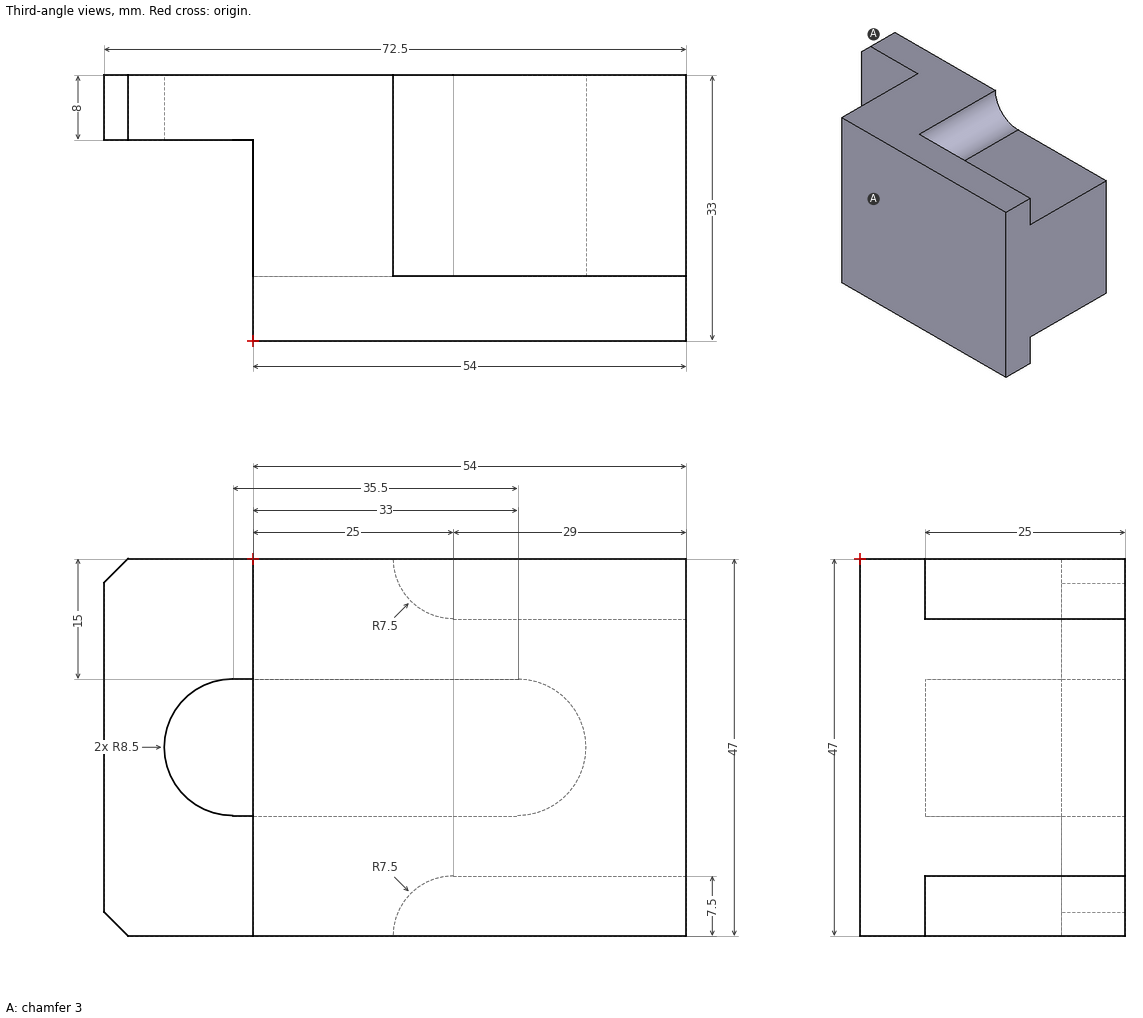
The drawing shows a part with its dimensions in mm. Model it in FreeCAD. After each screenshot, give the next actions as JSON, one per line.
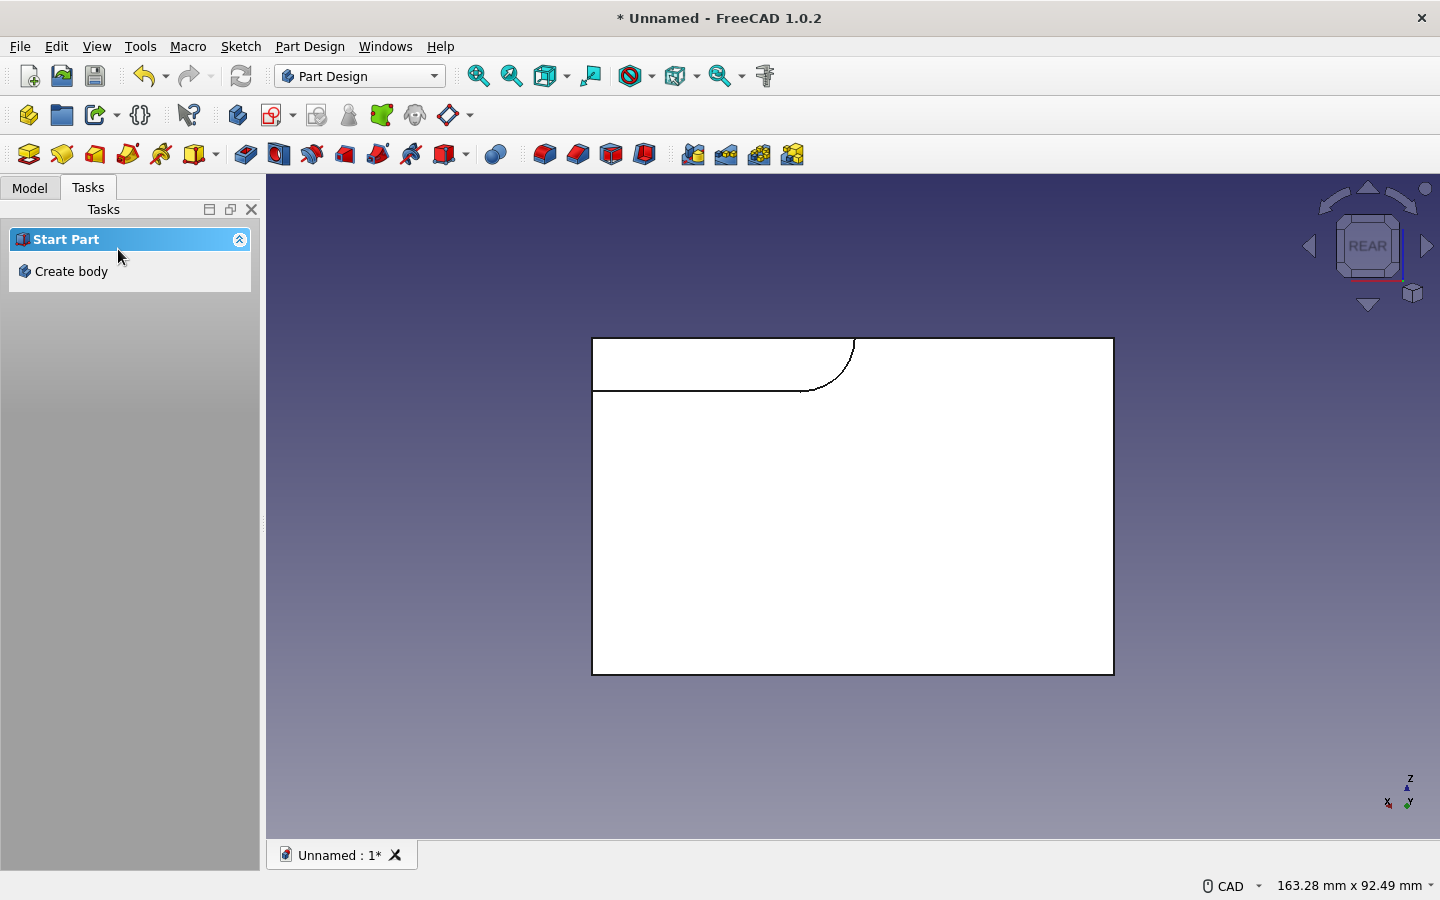
{"action": "left_click", "coordinate": [927, 505]}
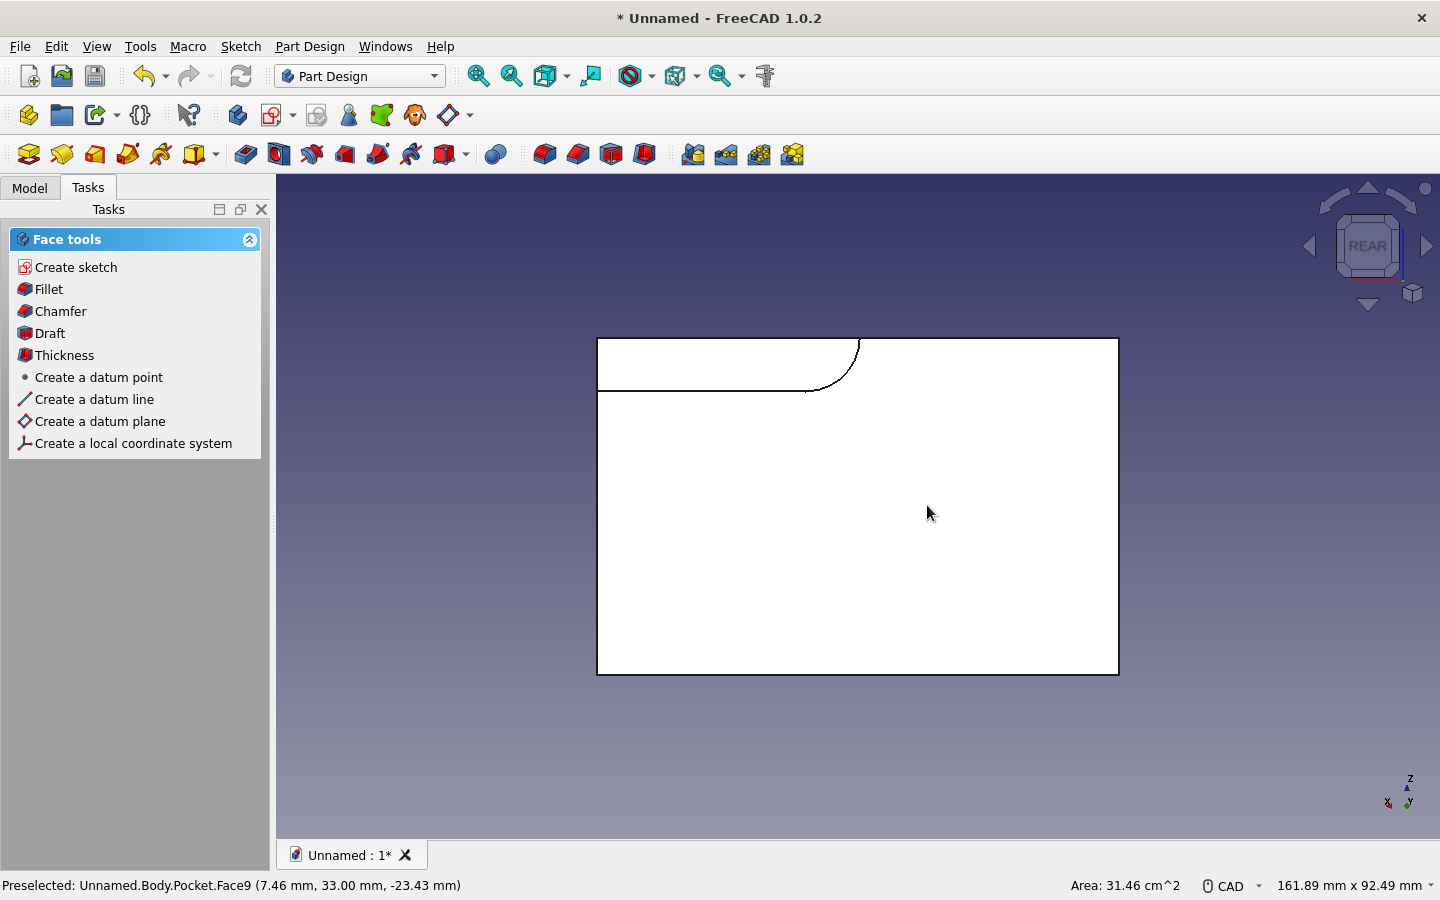
{"action": "left_click", "coordinate": [270, 116]}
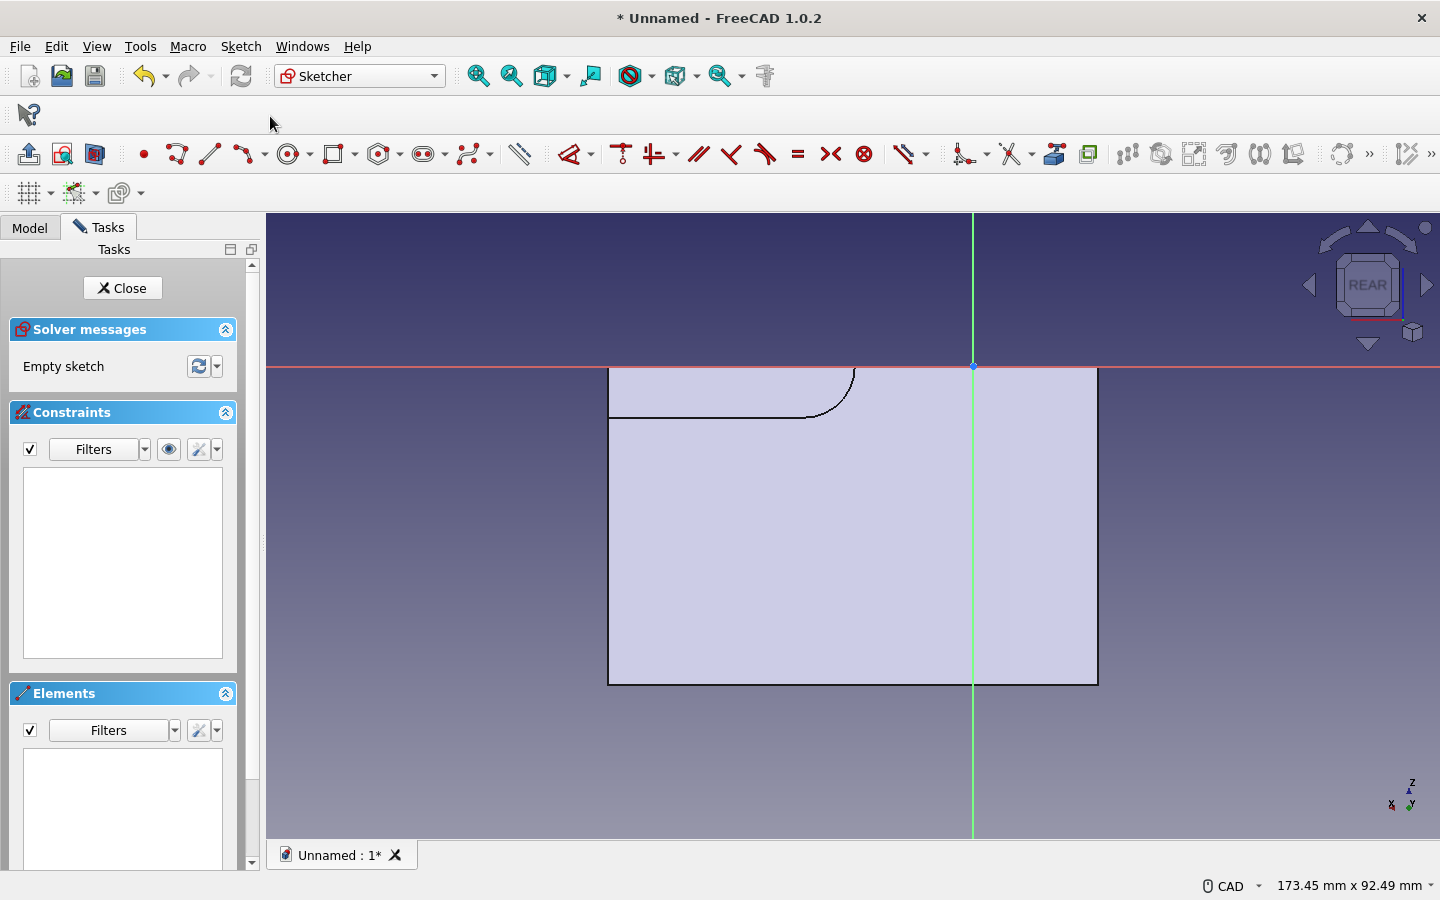
{"action": "key", "text": "g m"}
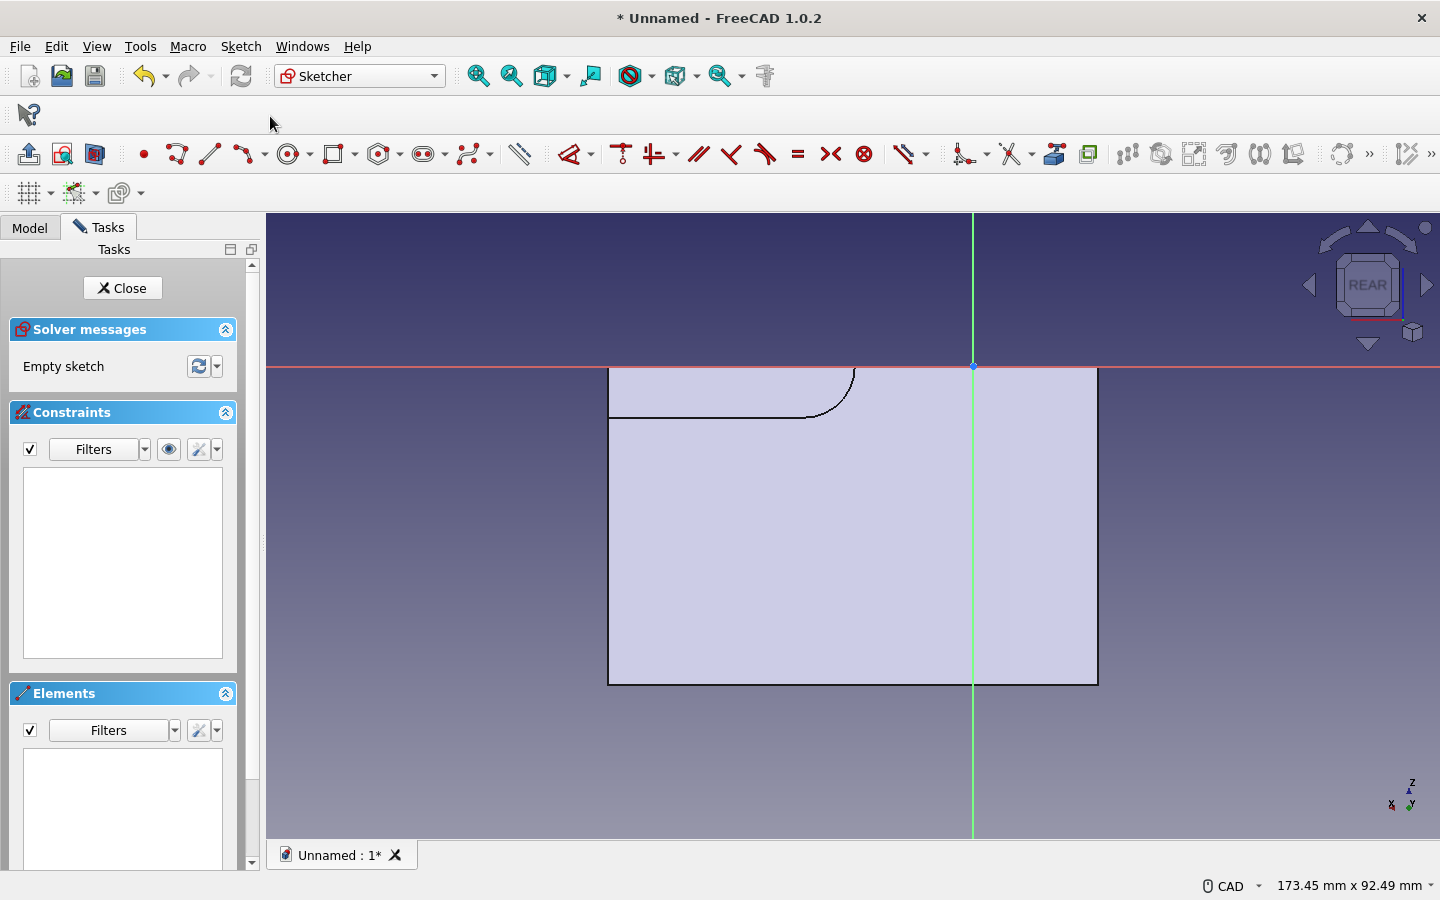
{"action": "left_click", "coordinate": [804, 634]}
{"action": "left_click", "coordinate": [608, 634]}
{"action": "left_click", "coordinate": [608, 685]}
{"action": "left_click", "coordinate": [855, 685]}
{"action": "right_click", "coordinate": [855, 685]}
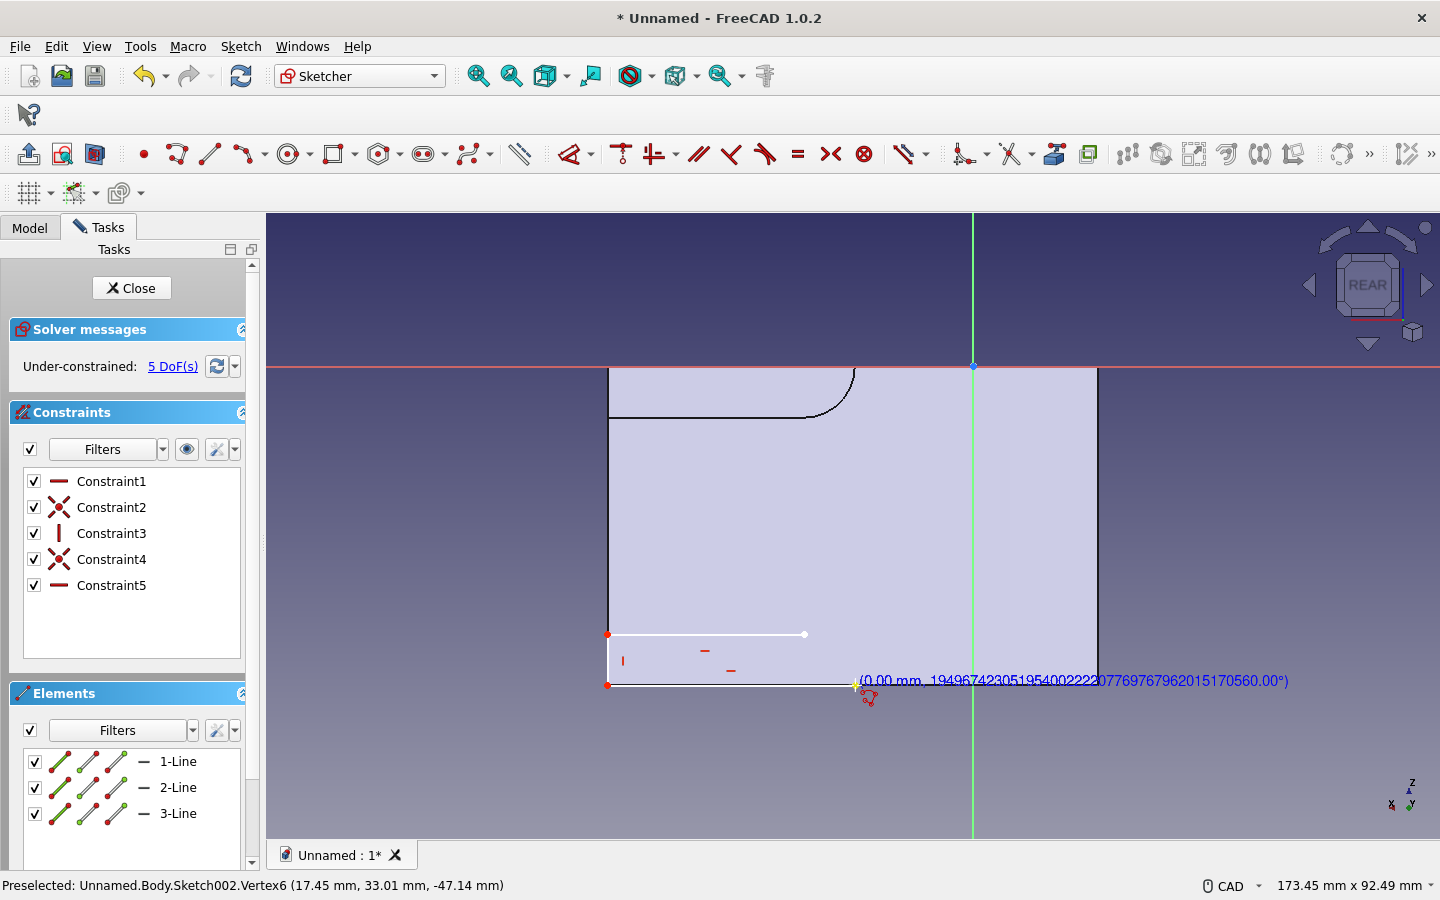
{"action": "key", "text": "g 3 a"}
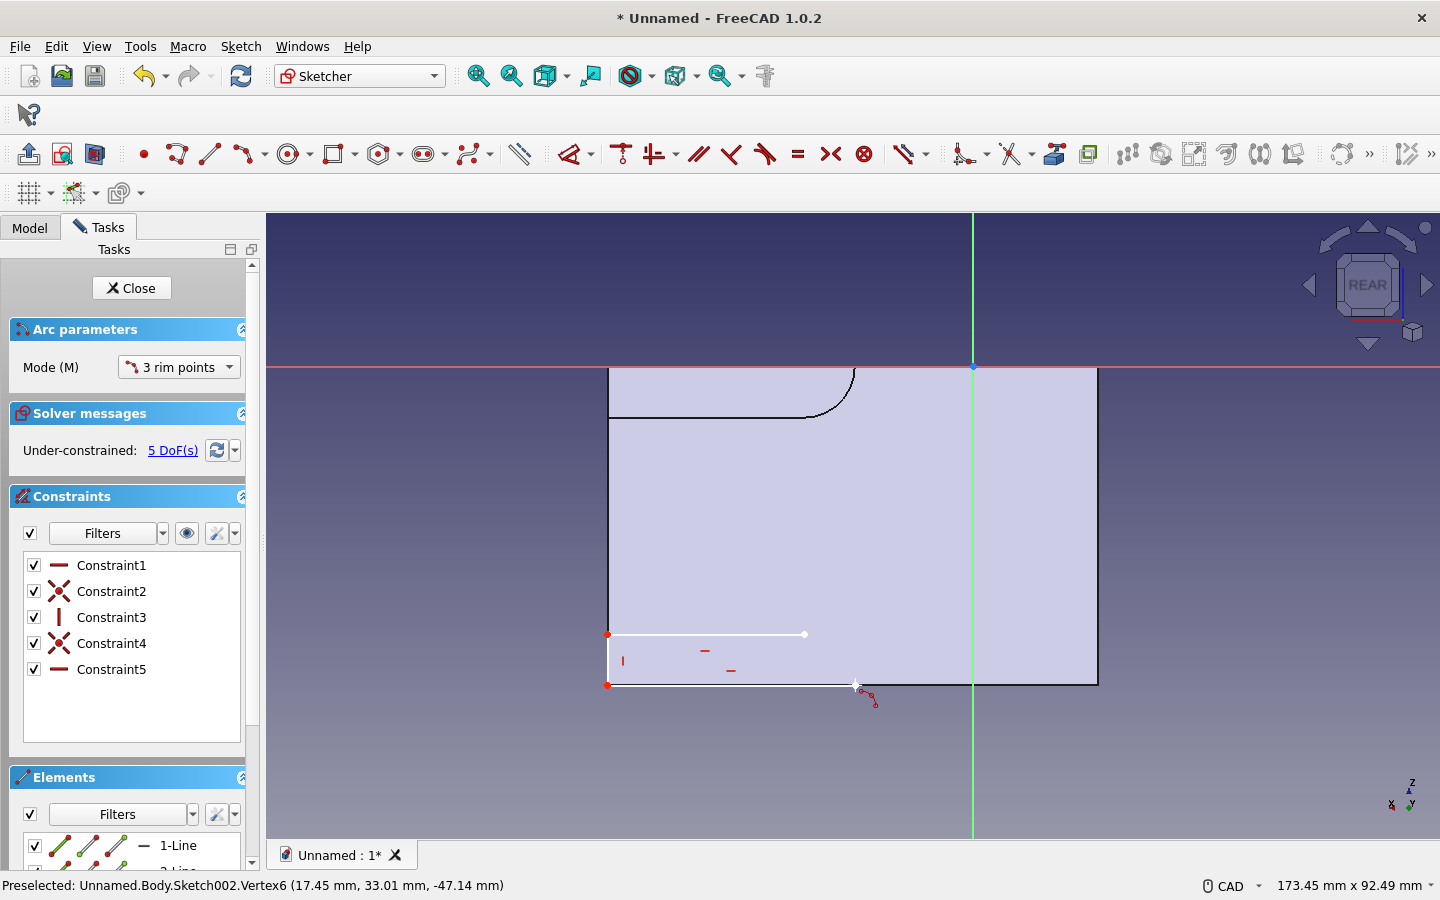
{"action": "left_click", "coordinate": [855, 686]}
{"action": "left_click", "coordinate": [804, 635]}
{"action": "left_click", "coordinate": [840, 649]}
{"action": "key", "text": "Escape"}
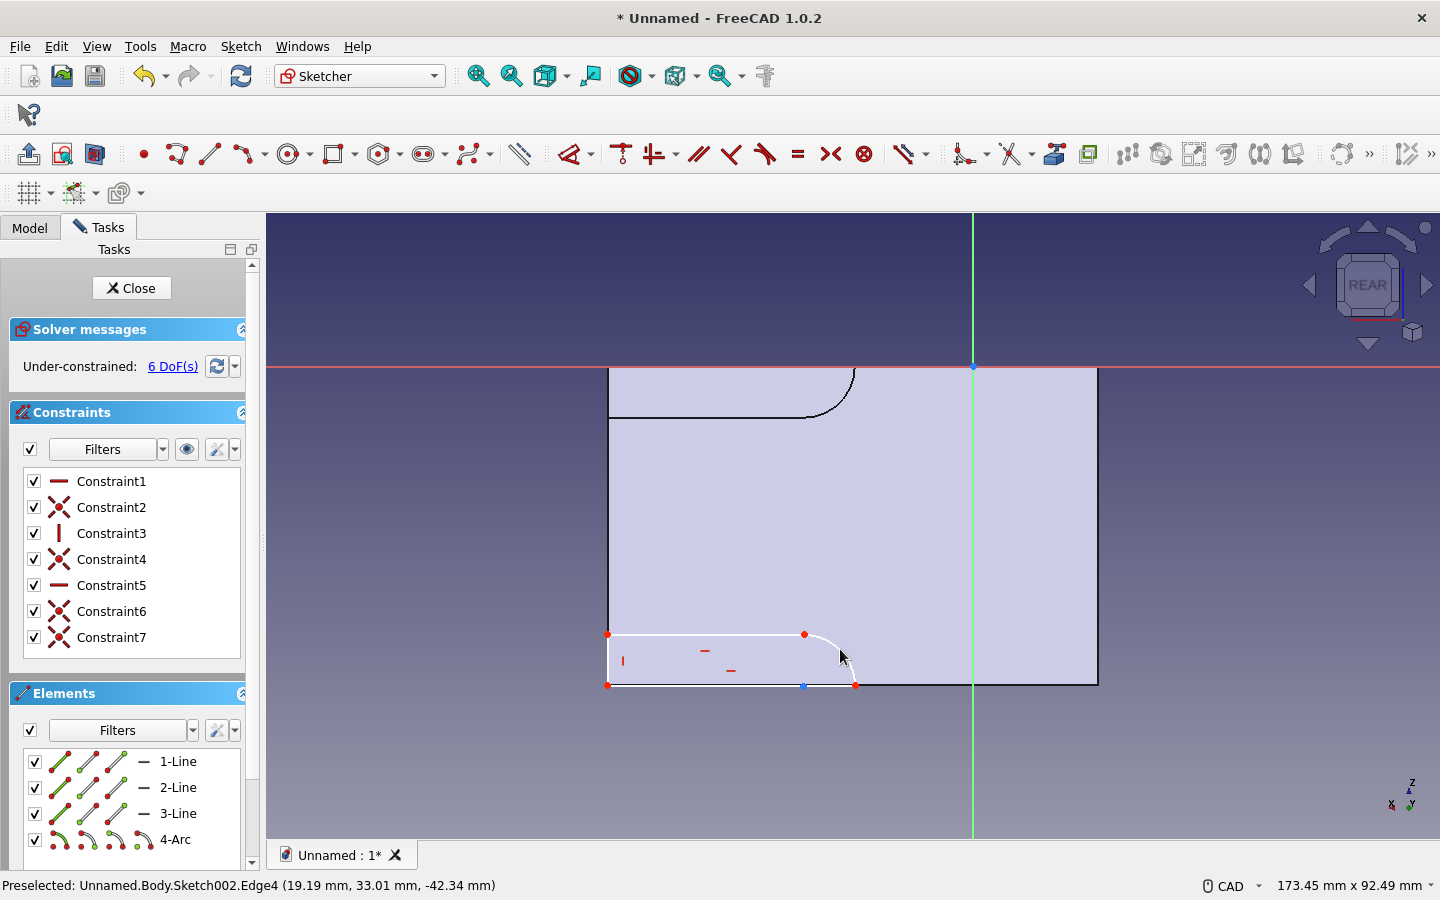
{"action": "left_click", "coordinate": [745, 635]}